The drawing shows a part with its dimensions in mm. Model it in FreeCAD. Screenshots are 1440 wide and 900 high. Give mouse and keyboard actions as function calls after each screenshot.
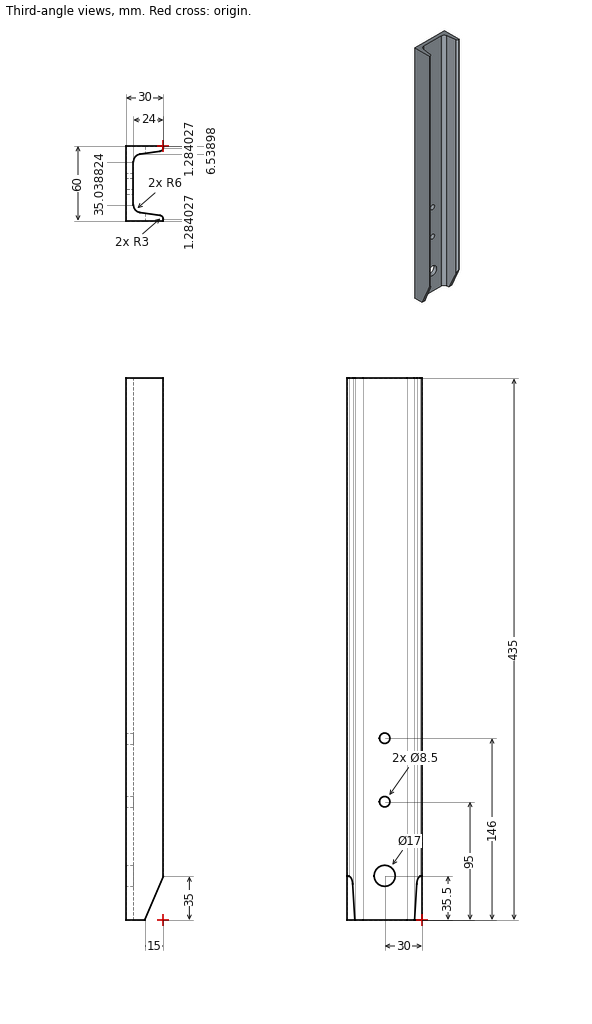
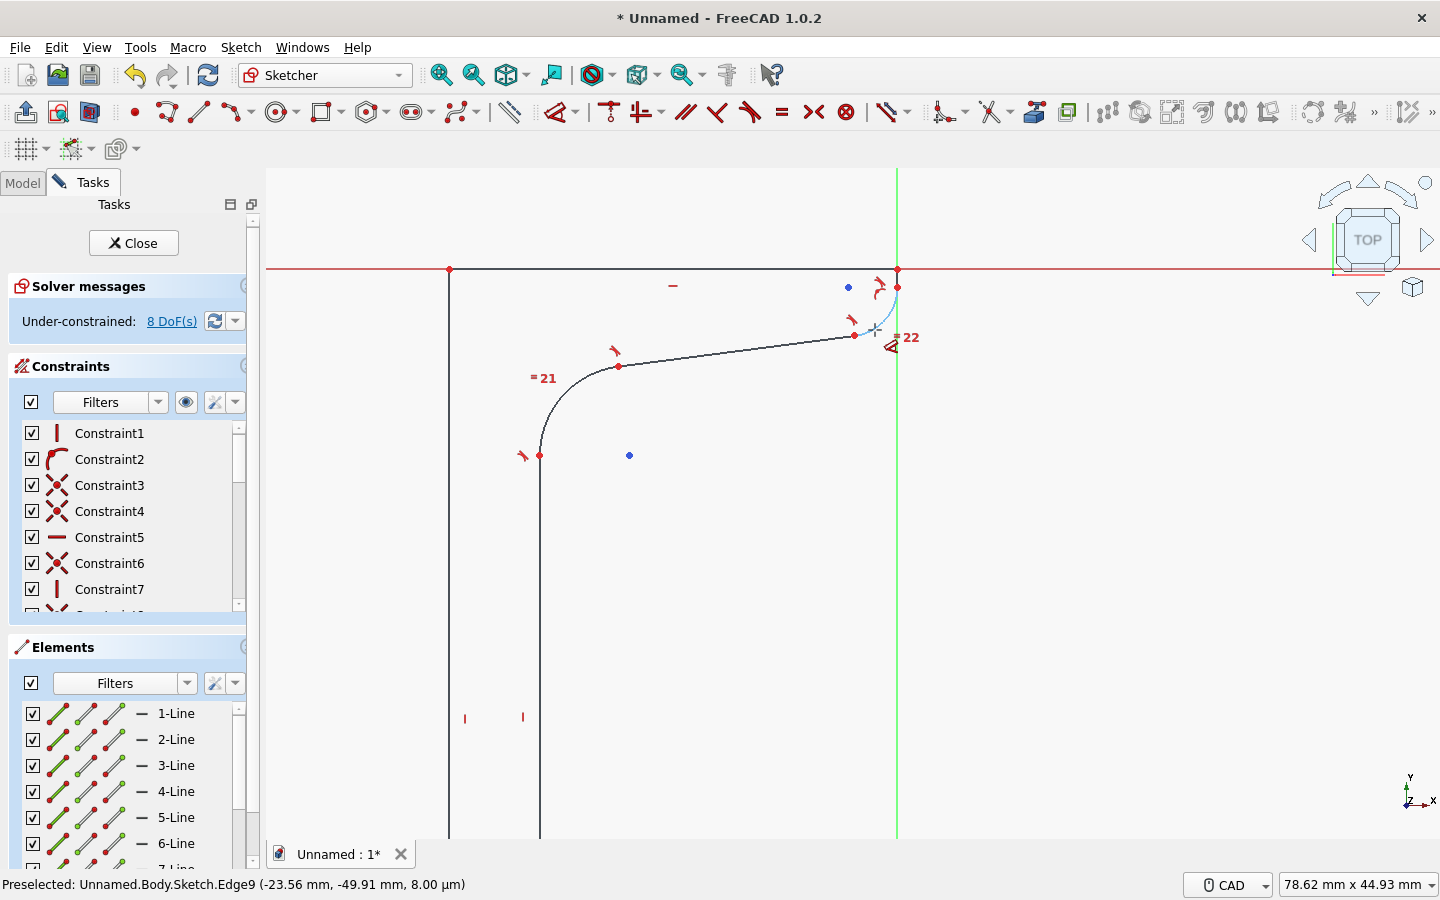
click(874, 329)
click(852, 368)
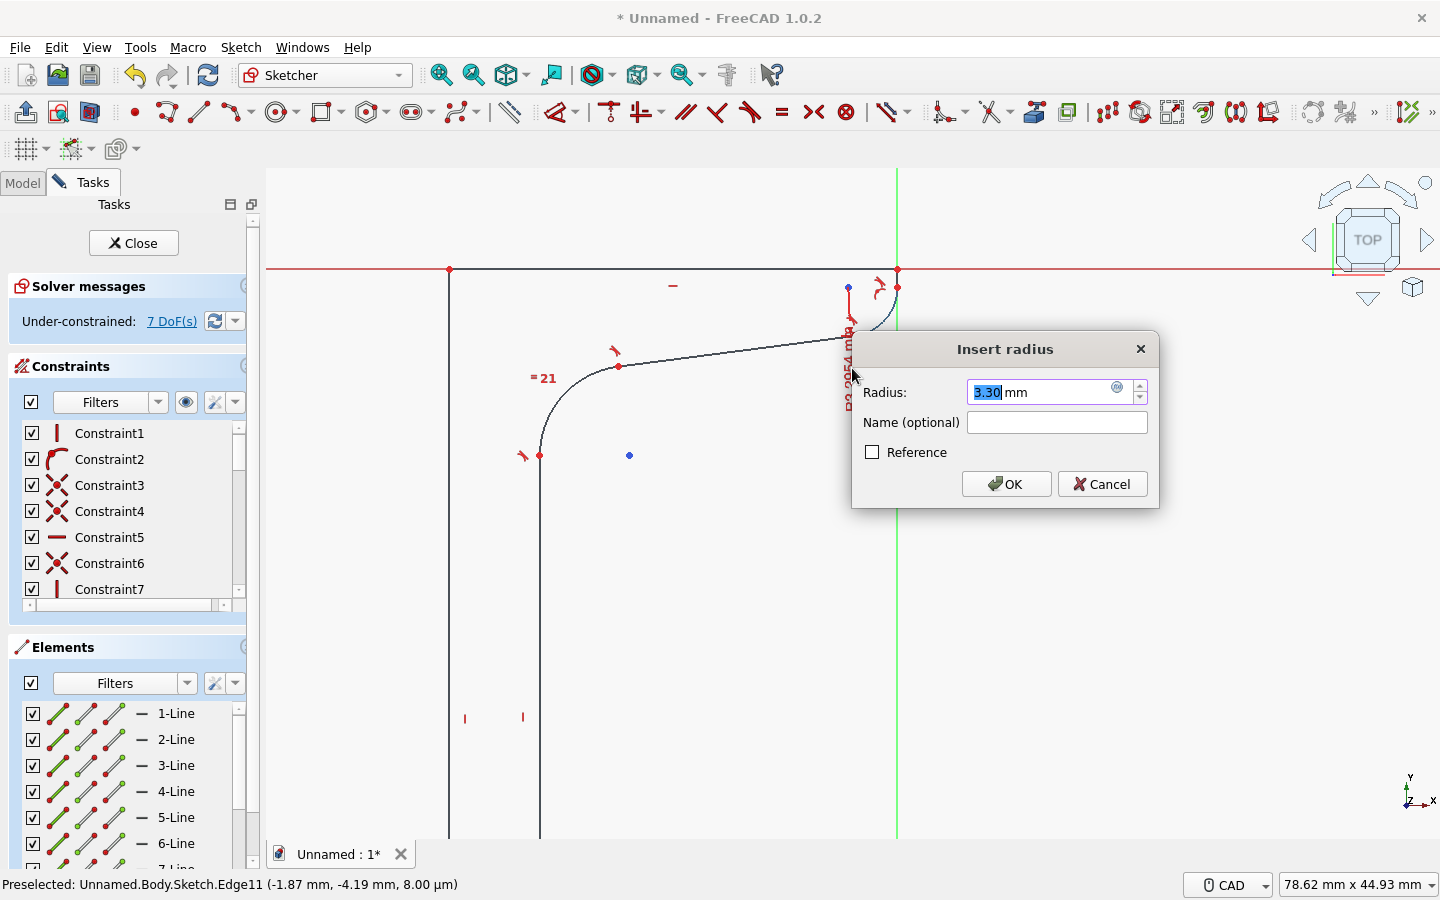
text(3)
key(Return)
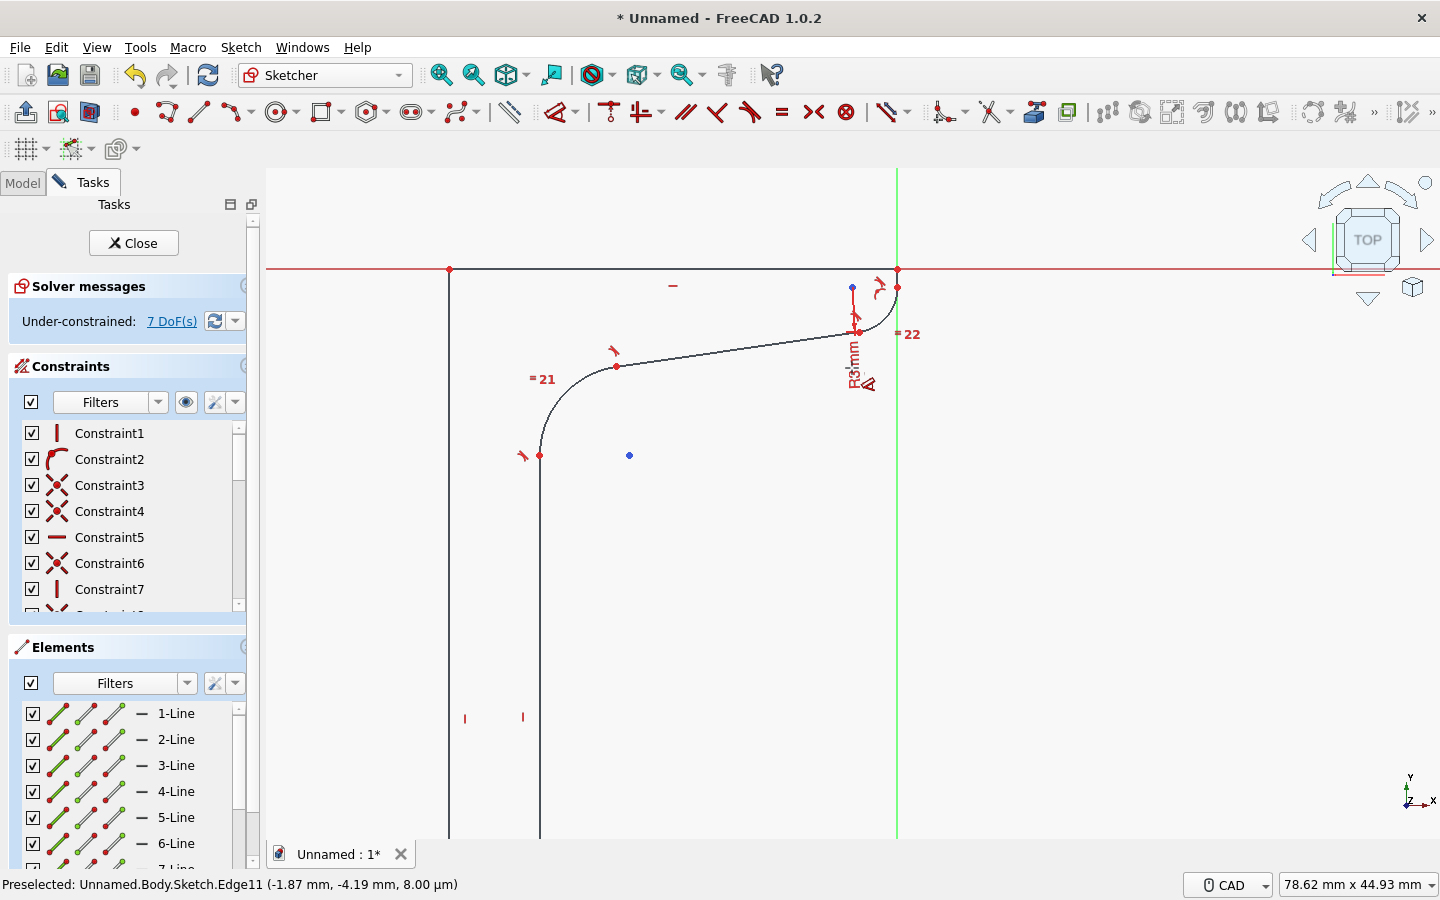
click(763, 269)
click(673, 235)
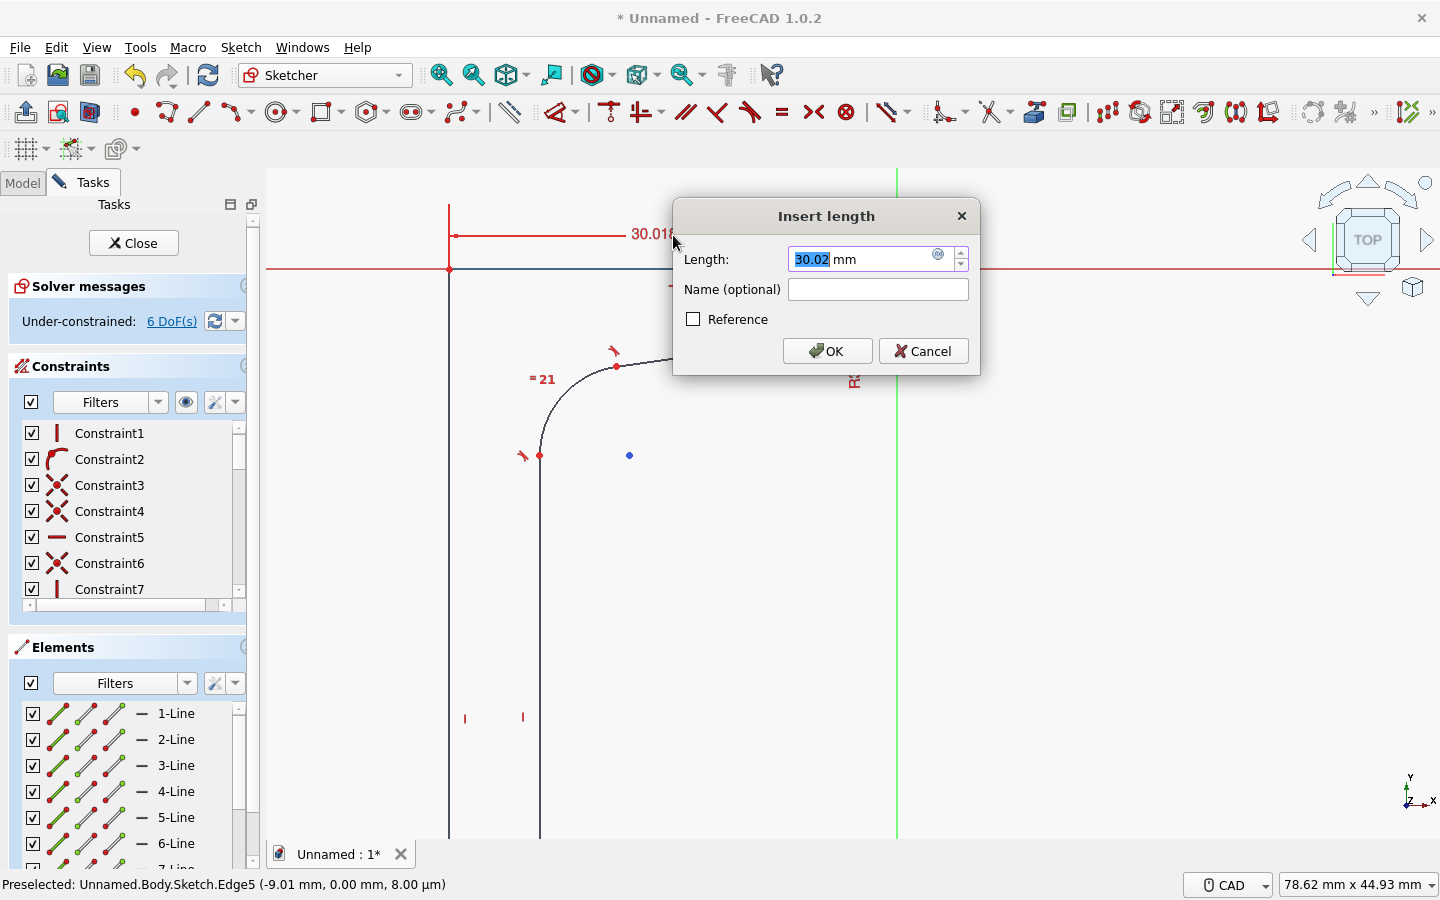
text(30)
key(Return)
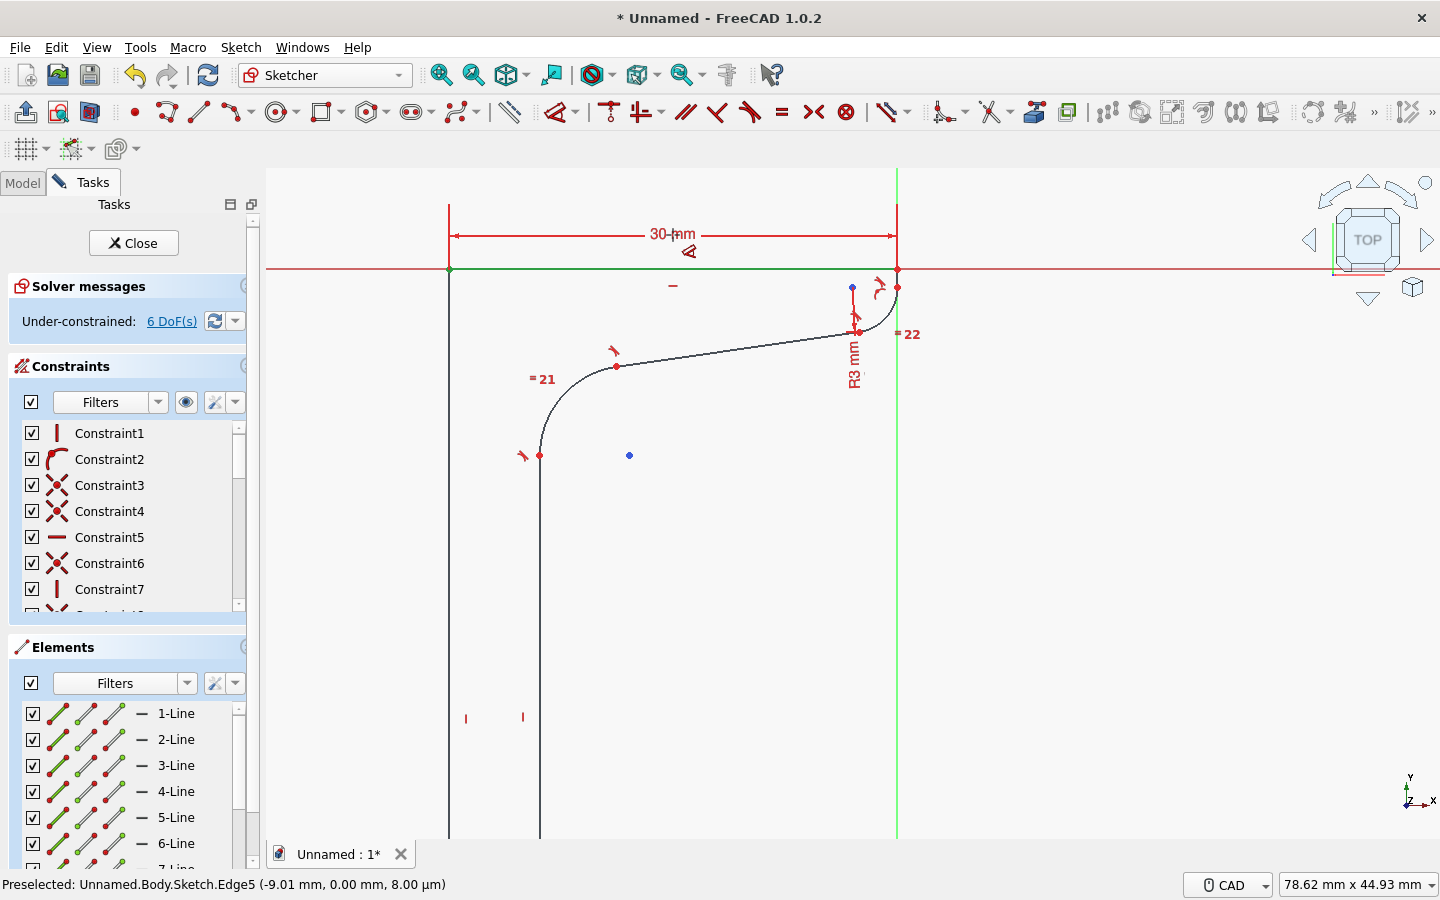
click(449, 539)
click(415, 540)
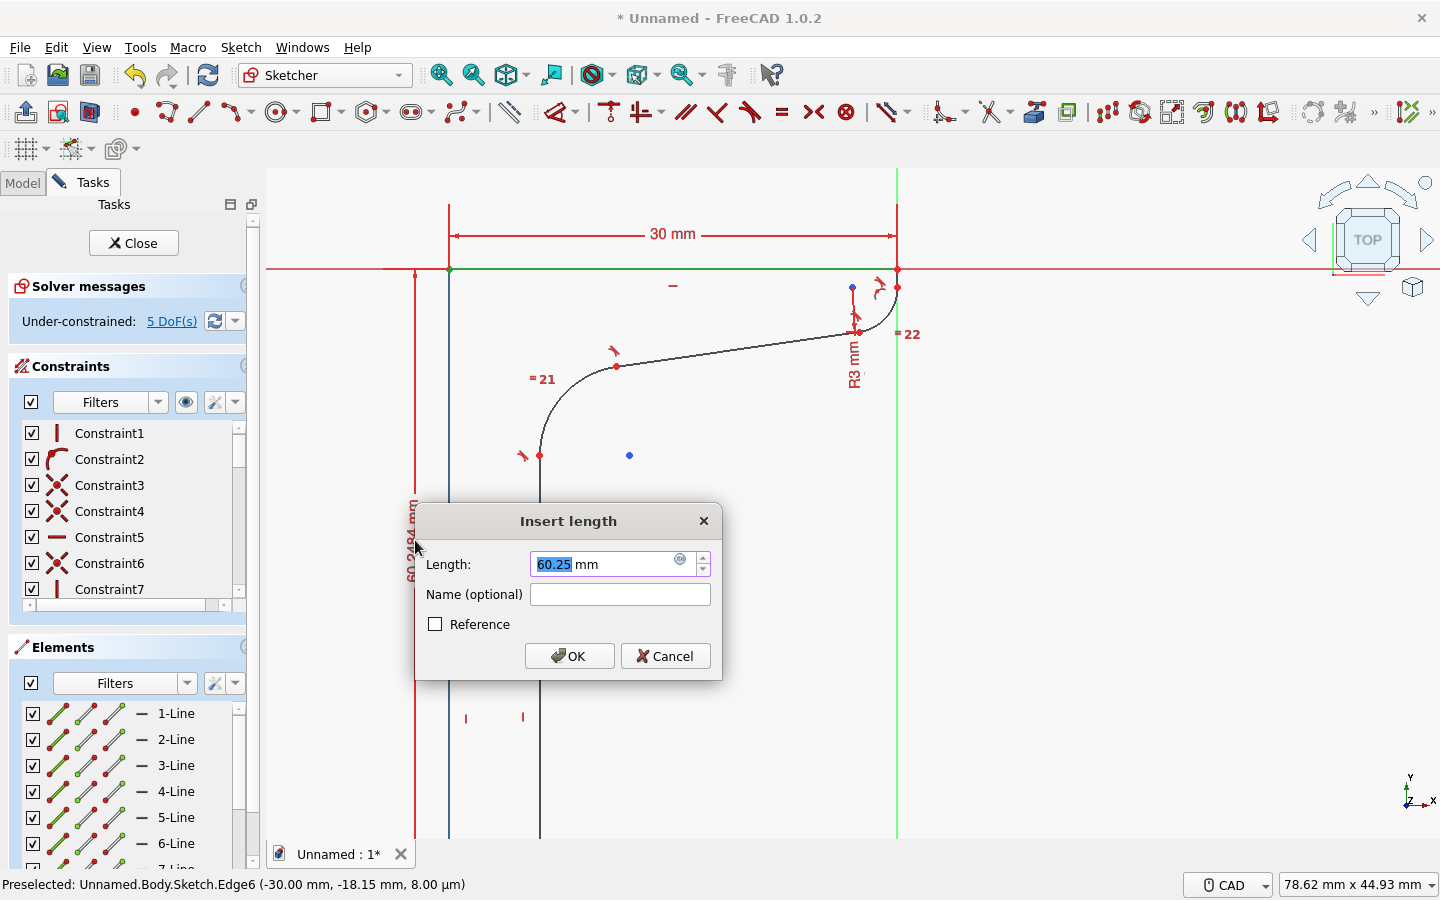
text(60)
key(Return)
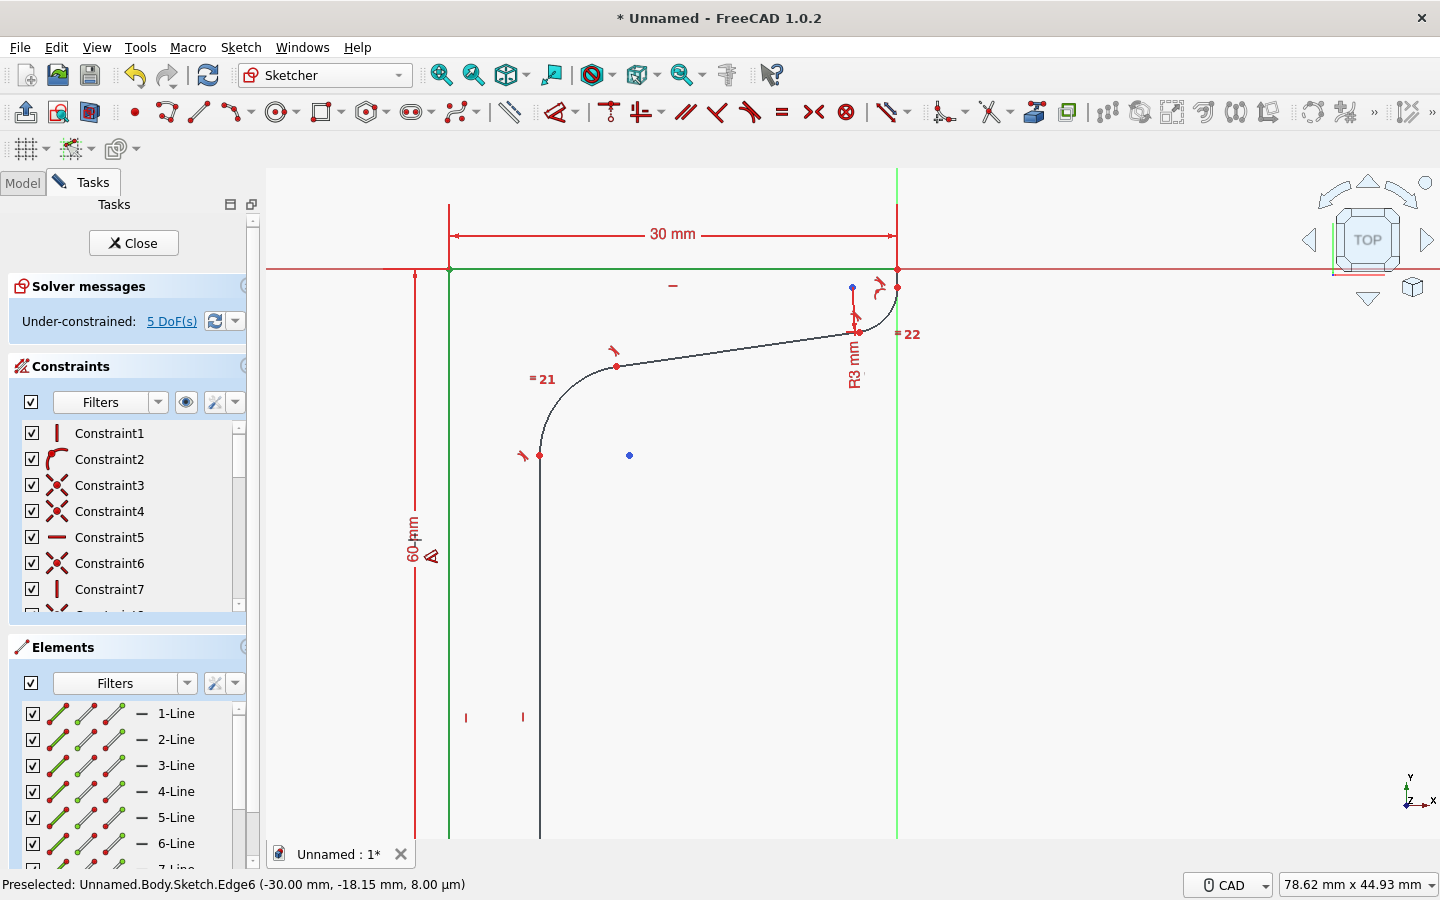
scroll(875, 329, down, 4)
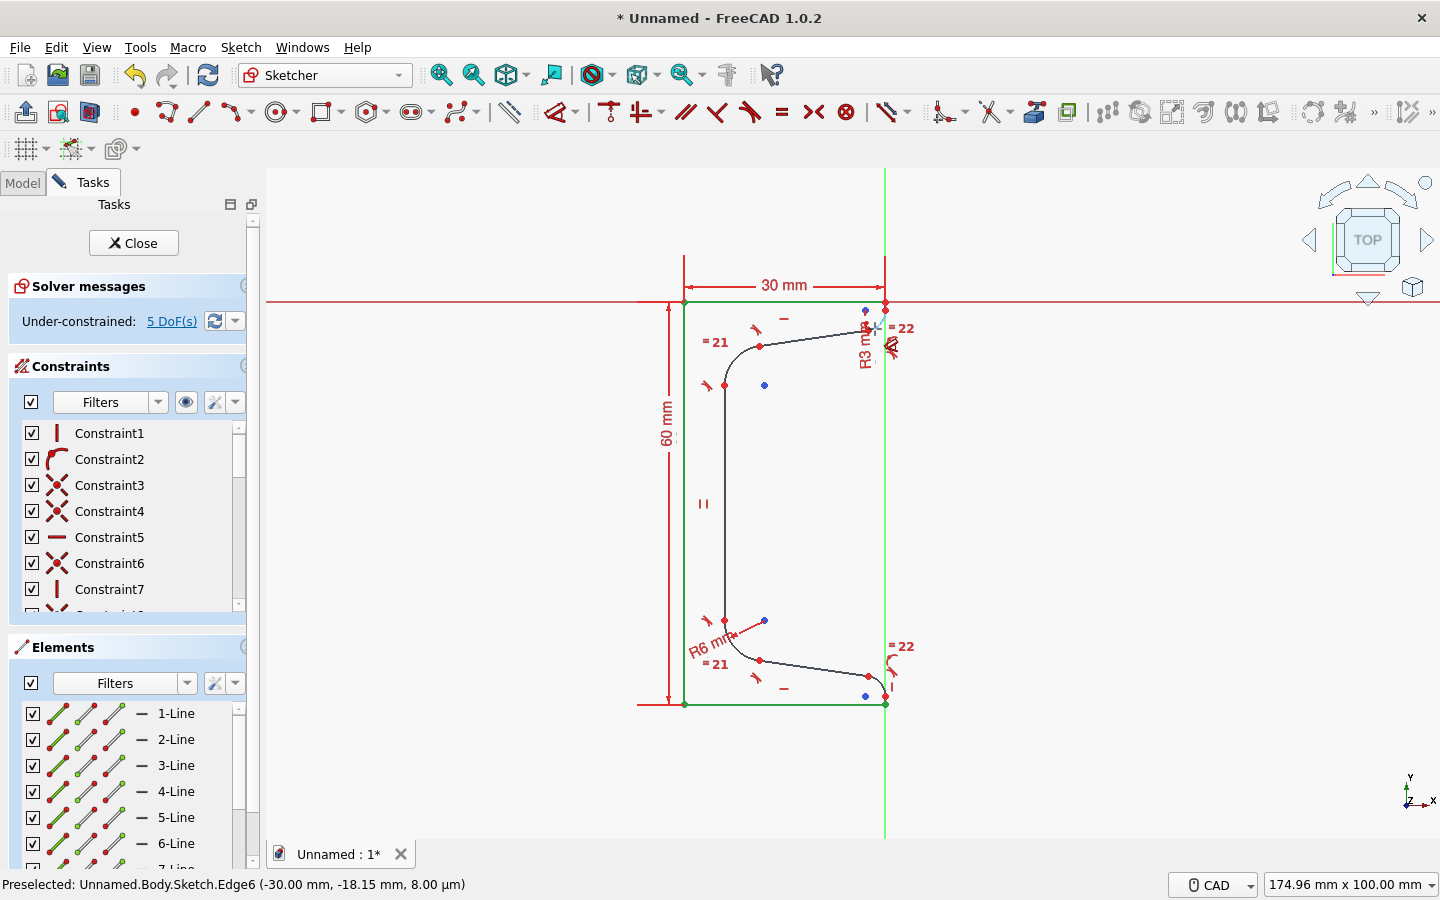
click(725, 621)
click(861, 268)